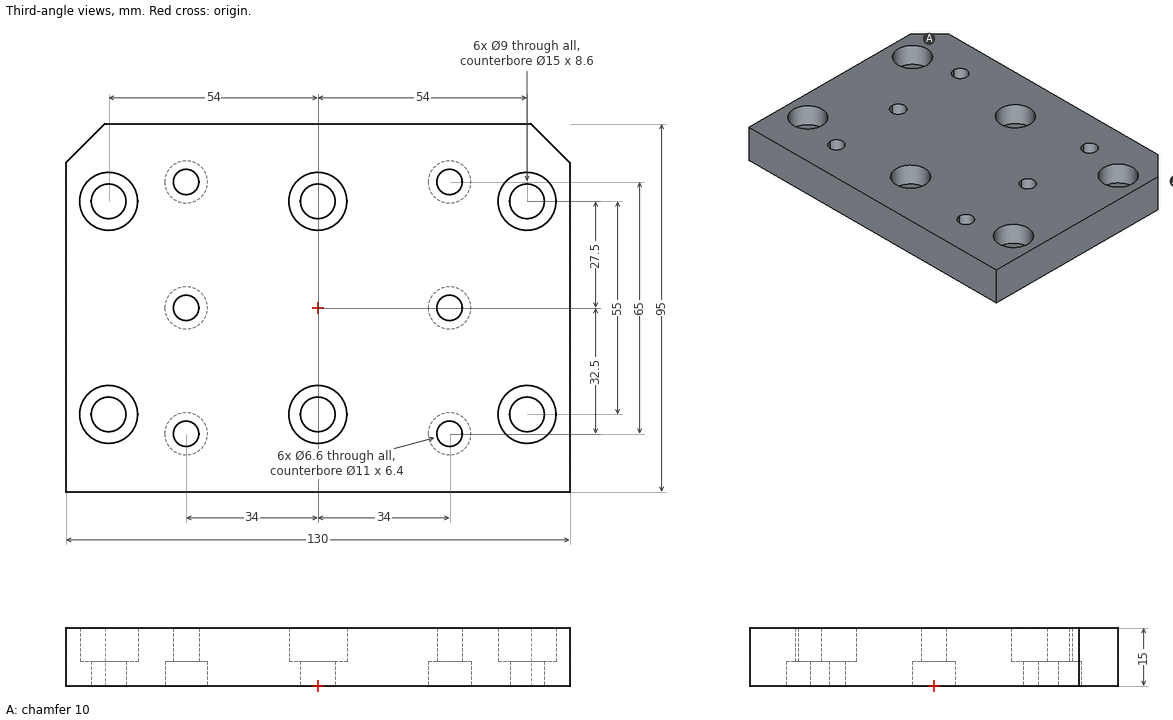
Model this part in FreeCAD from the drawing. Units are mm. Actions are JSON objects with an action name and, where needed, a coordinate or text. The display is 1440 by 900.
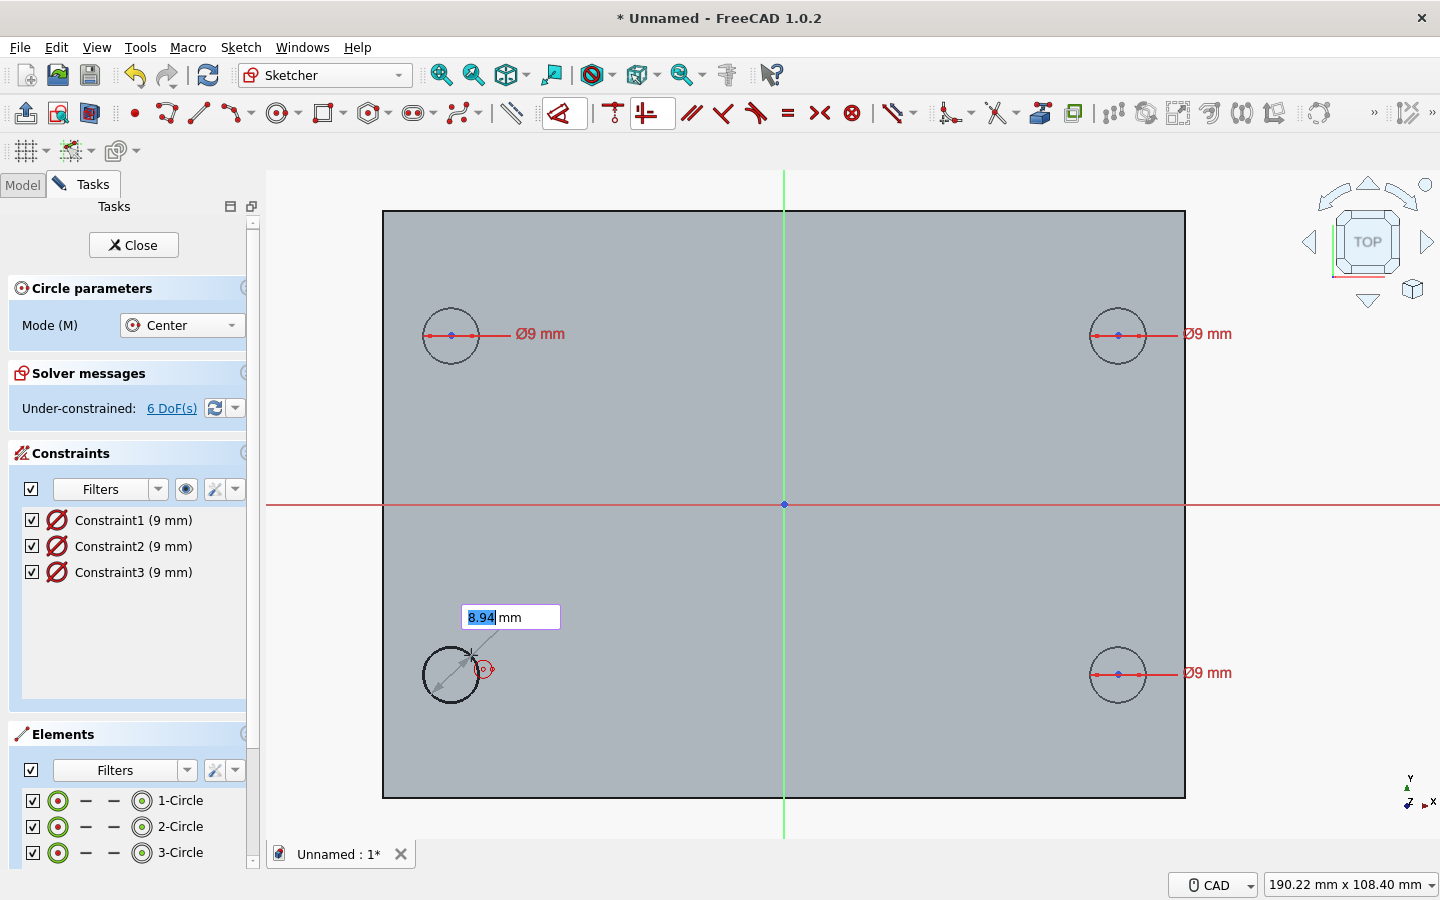
{"action": "type", "text": "9"}
{"action": "key", "text": "Return"}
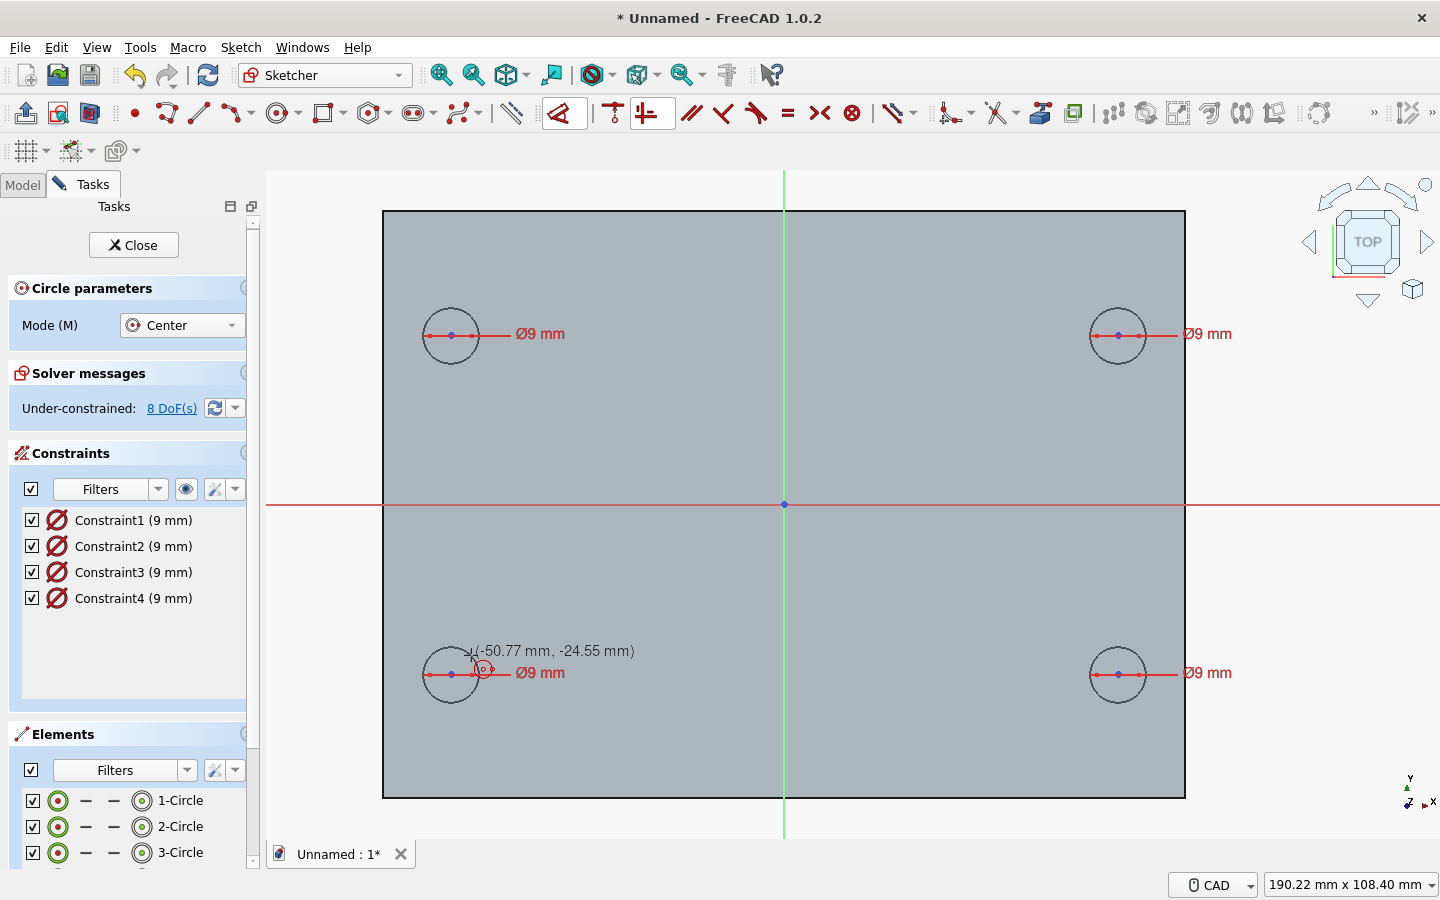
{"action": "left_click", "coordinate": [784, 335]}
{"action": "mouse_move", "coordinate": [804, 315]}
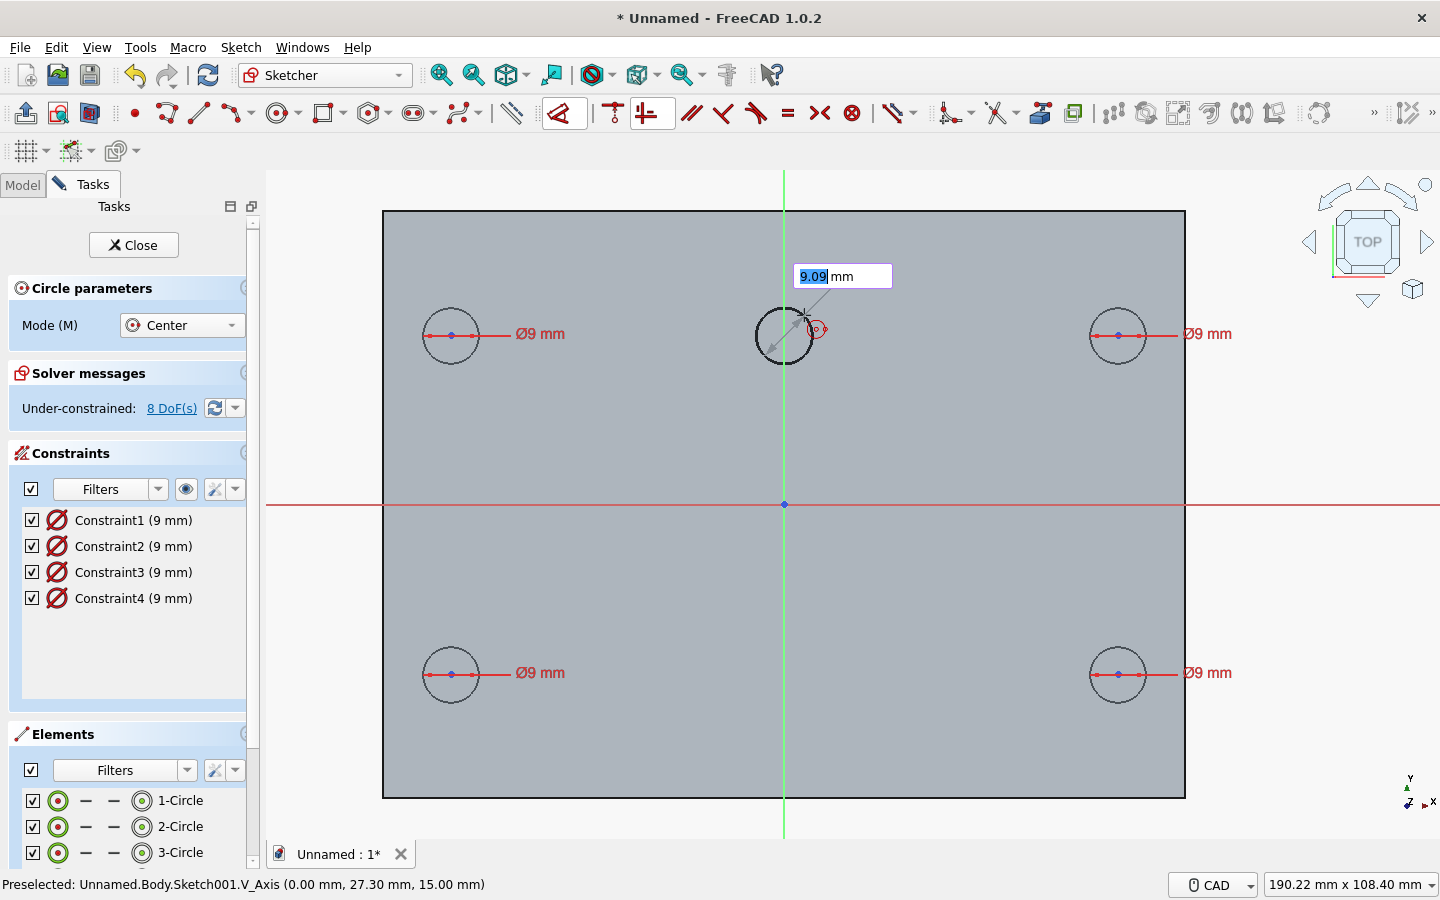
{"action": "type", "text": "9"}
{"action": "key", "text": "Return"}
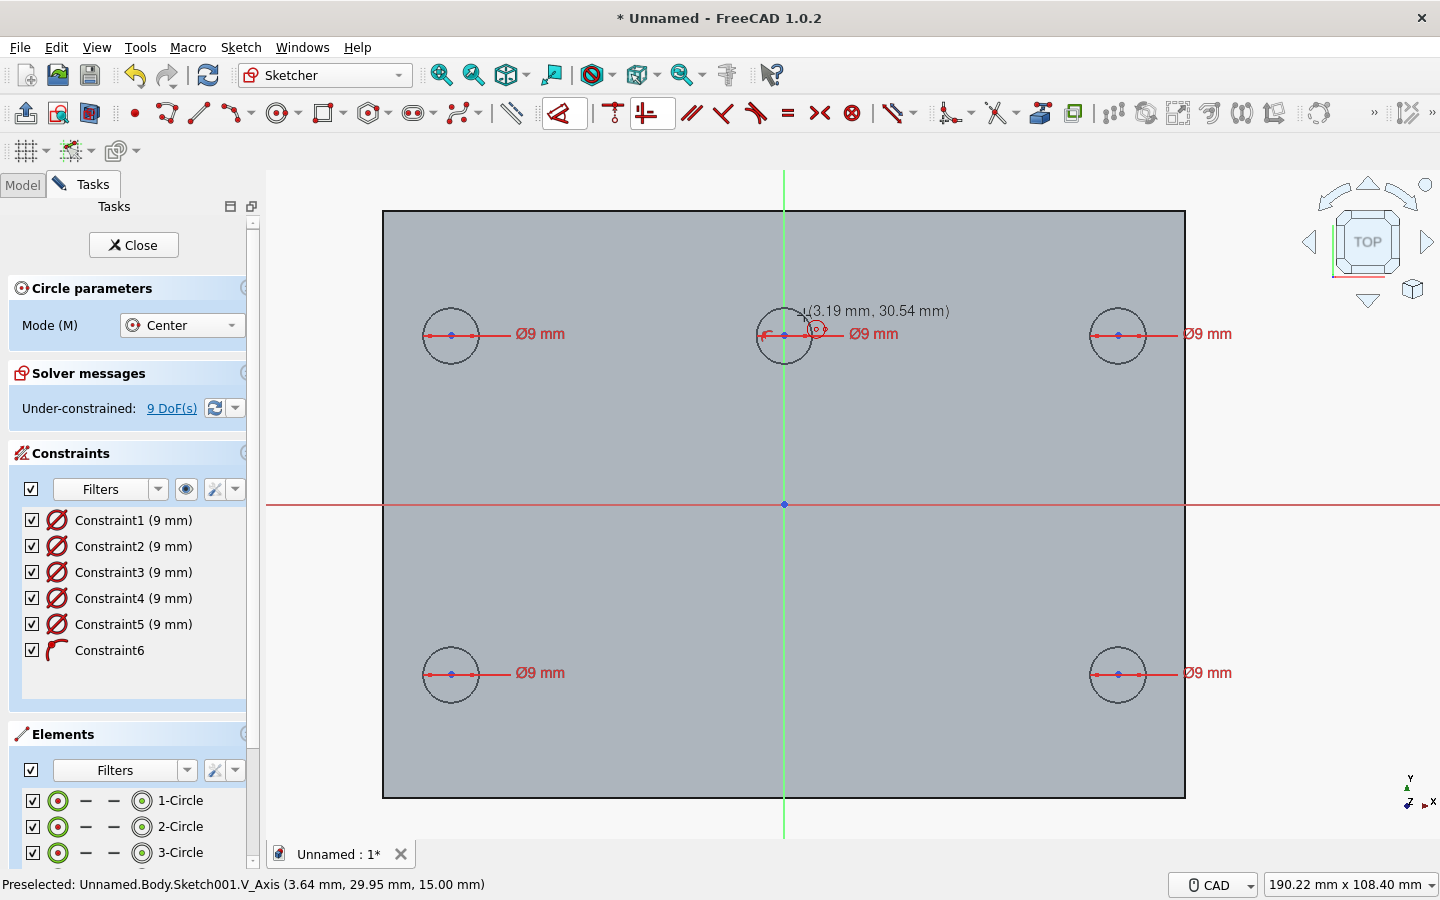
{"action": "left_click", "coordinate": [784, 674]}
{"action": "mouse_move", "coordinate": [804, 655]}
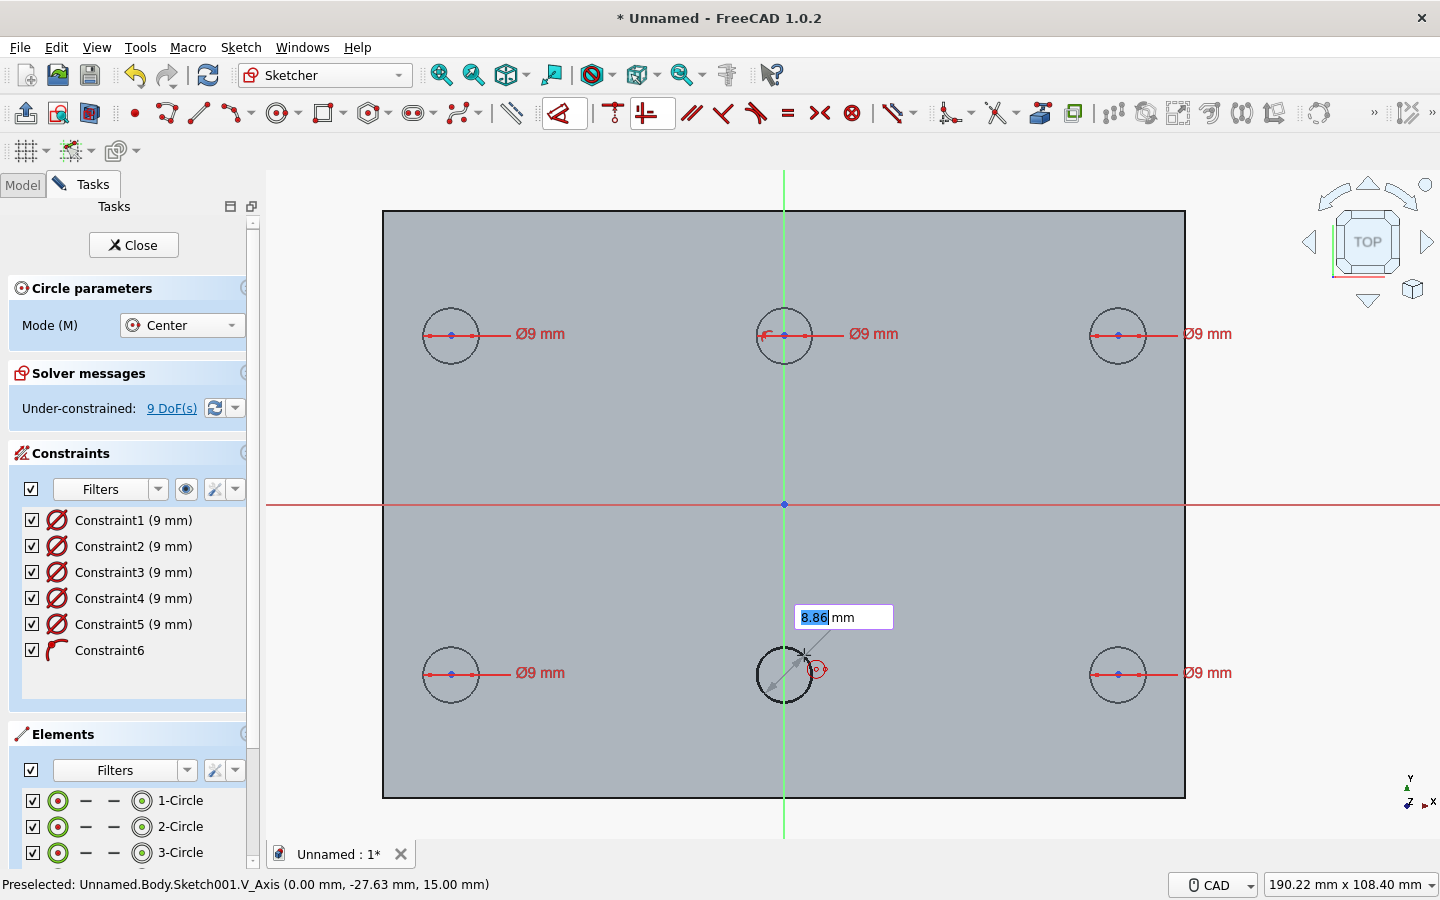
{"action": "type", "text": "9"}
{"action": "key", "text": "Return"}
{"action": "key", "text": "Escape"}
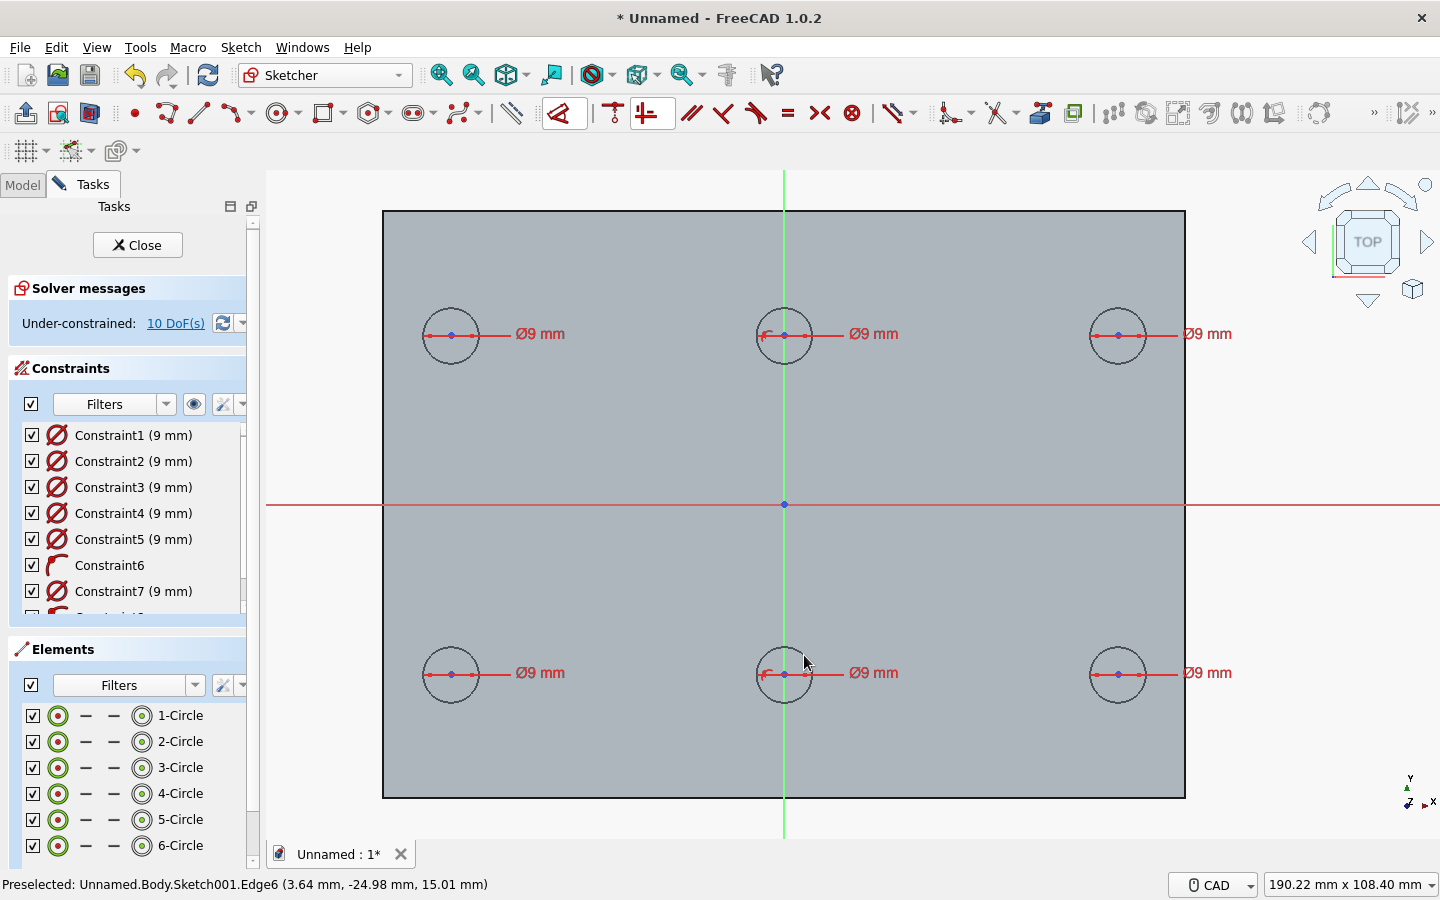
{"action": "left_click", "coordinate": [1118, 336]}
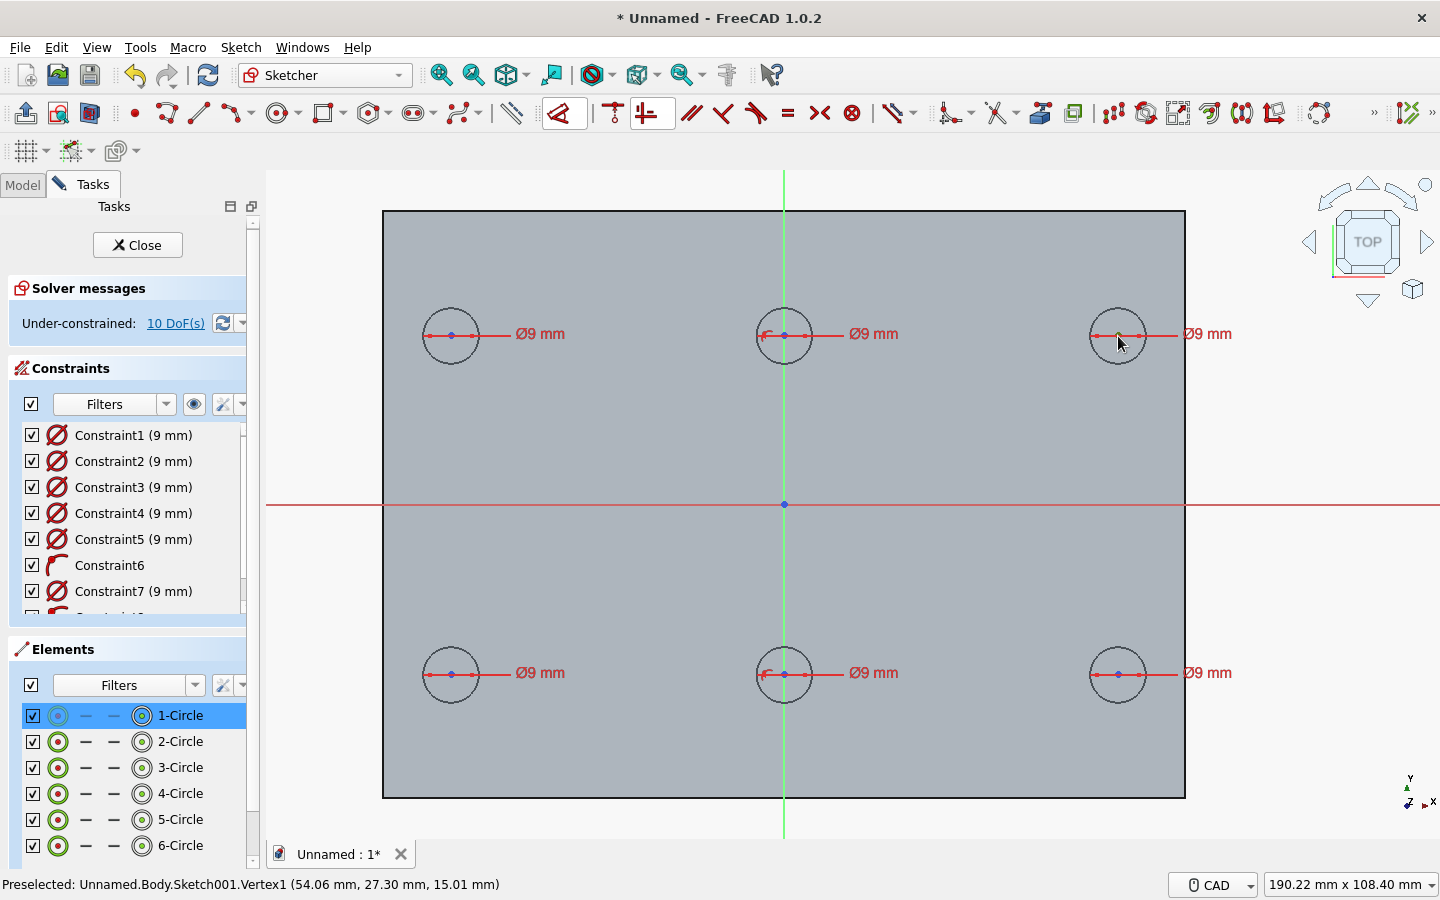
{"action": "left_click", "coordinate": [1118, 675]}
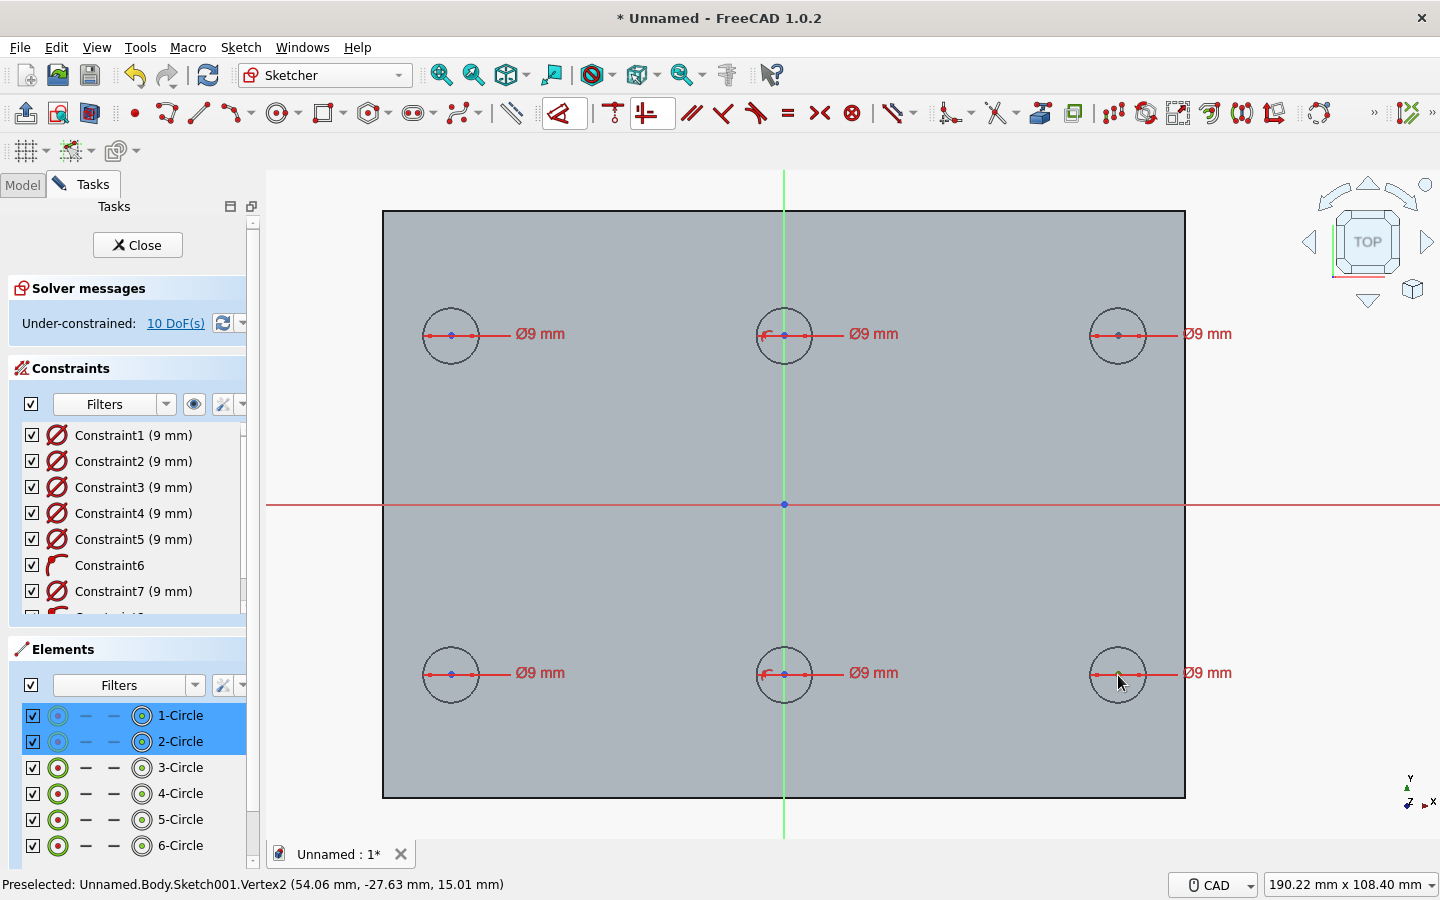
{"action": "key", "text": "v"}